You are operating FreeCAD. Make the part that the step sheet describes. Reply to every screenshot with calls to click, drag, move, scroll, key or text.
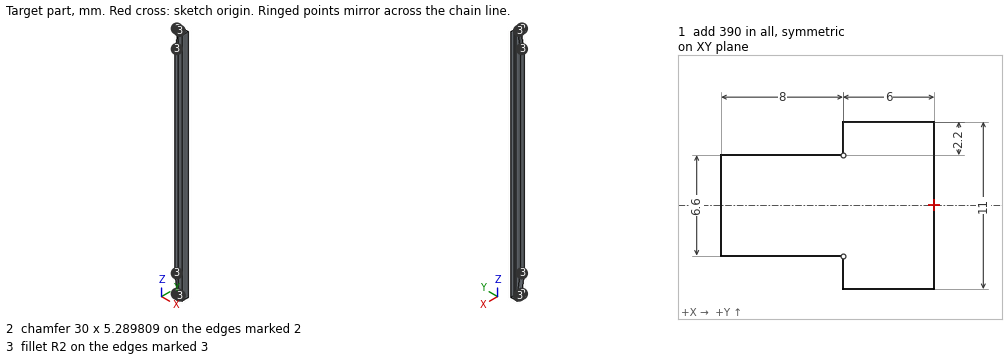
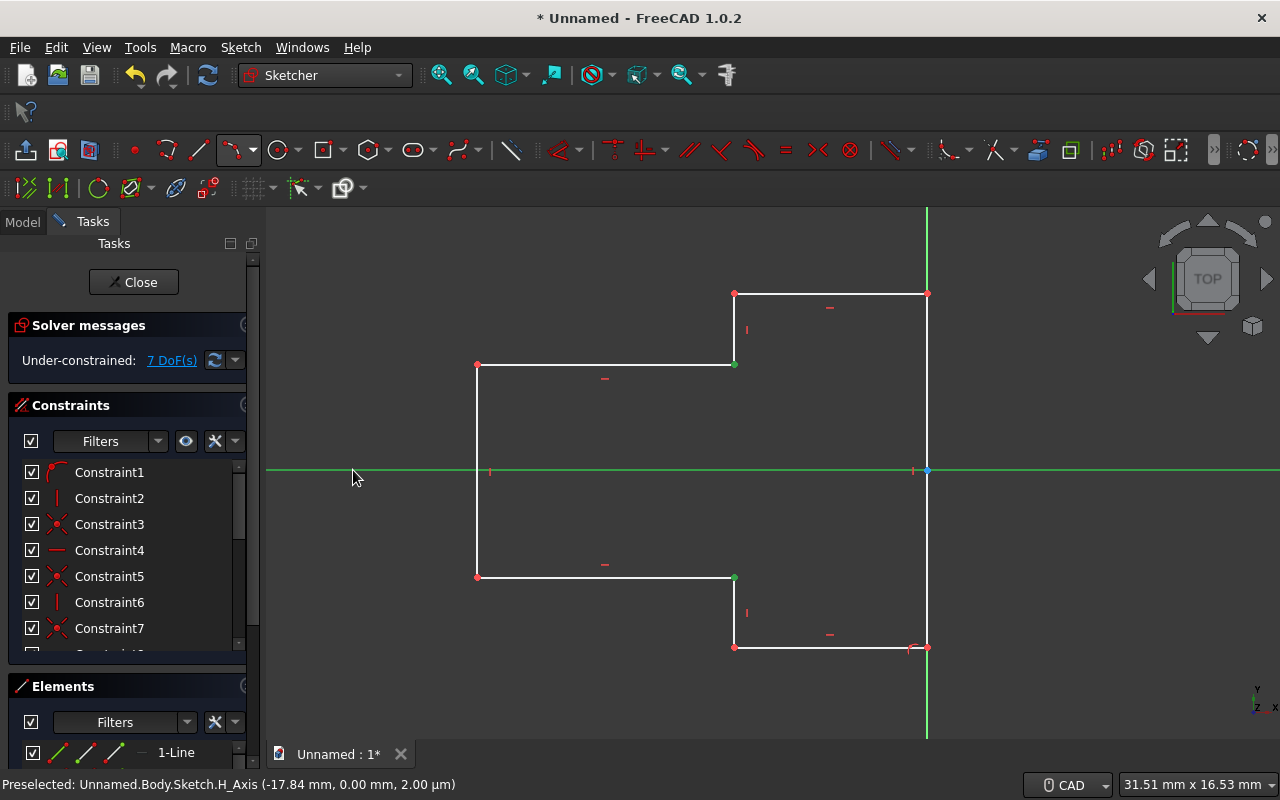
click(818, 150)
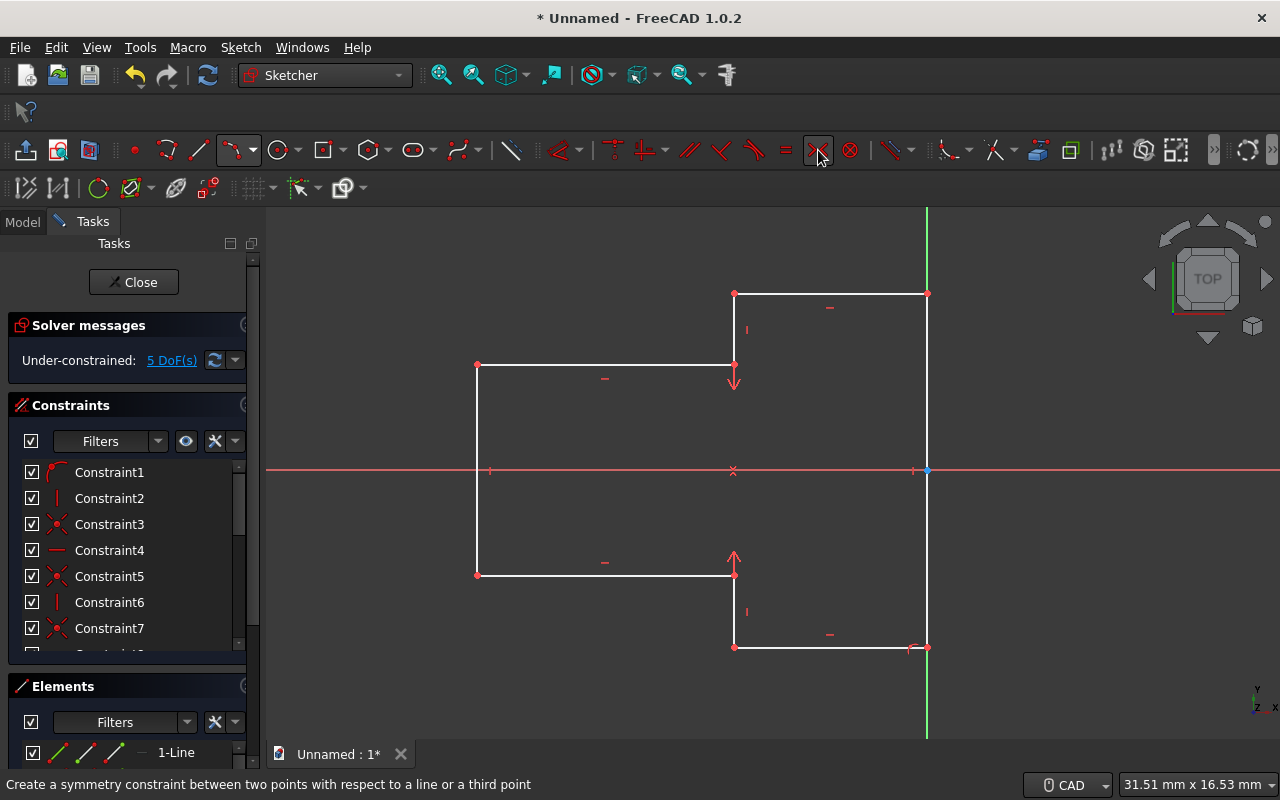
click(558, 150)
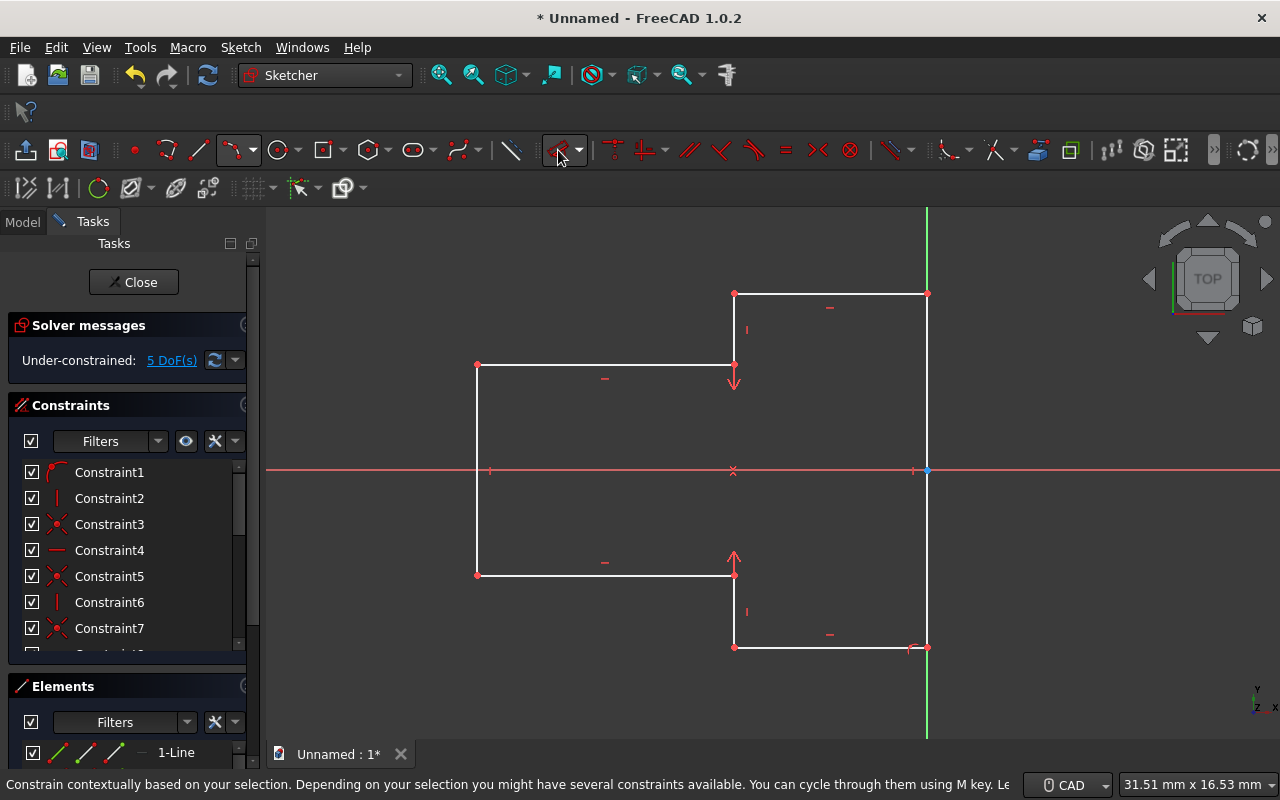
click(869, 294)
click(831, 260)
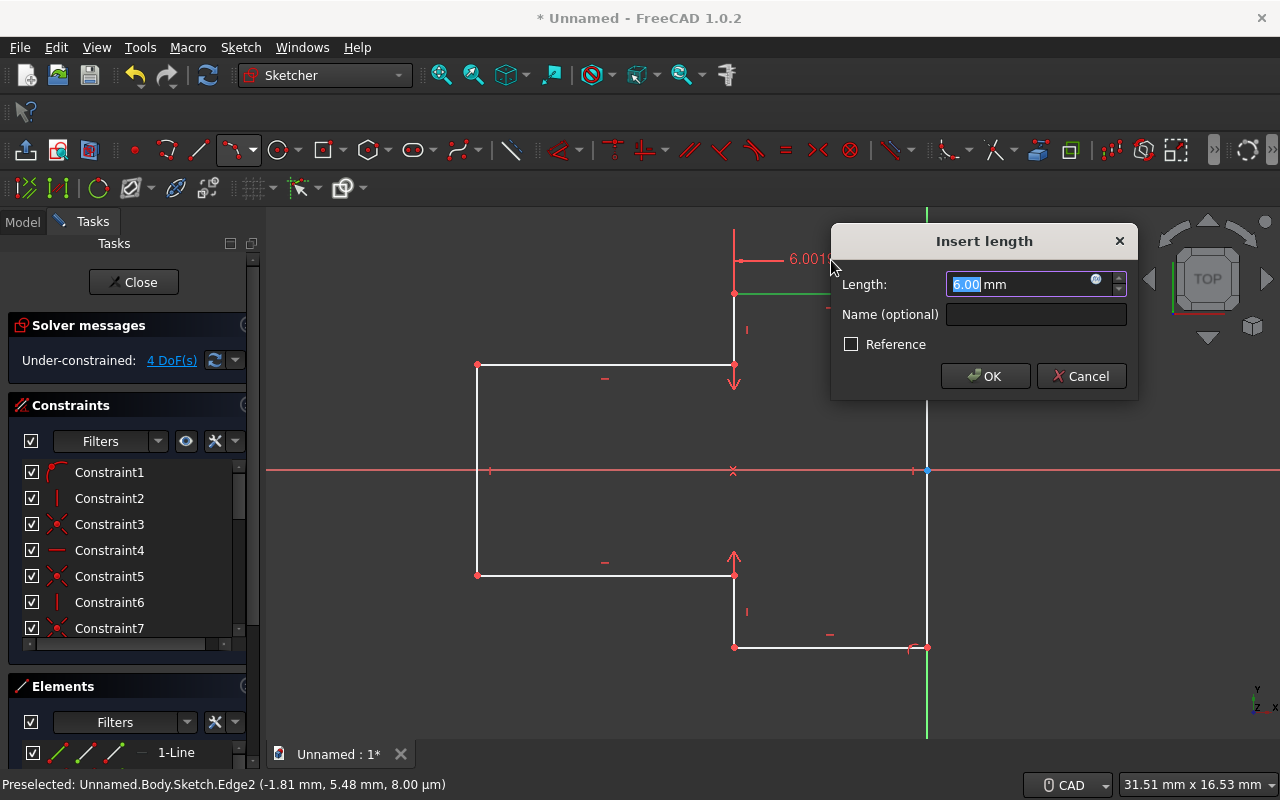
text(6)
key(Return)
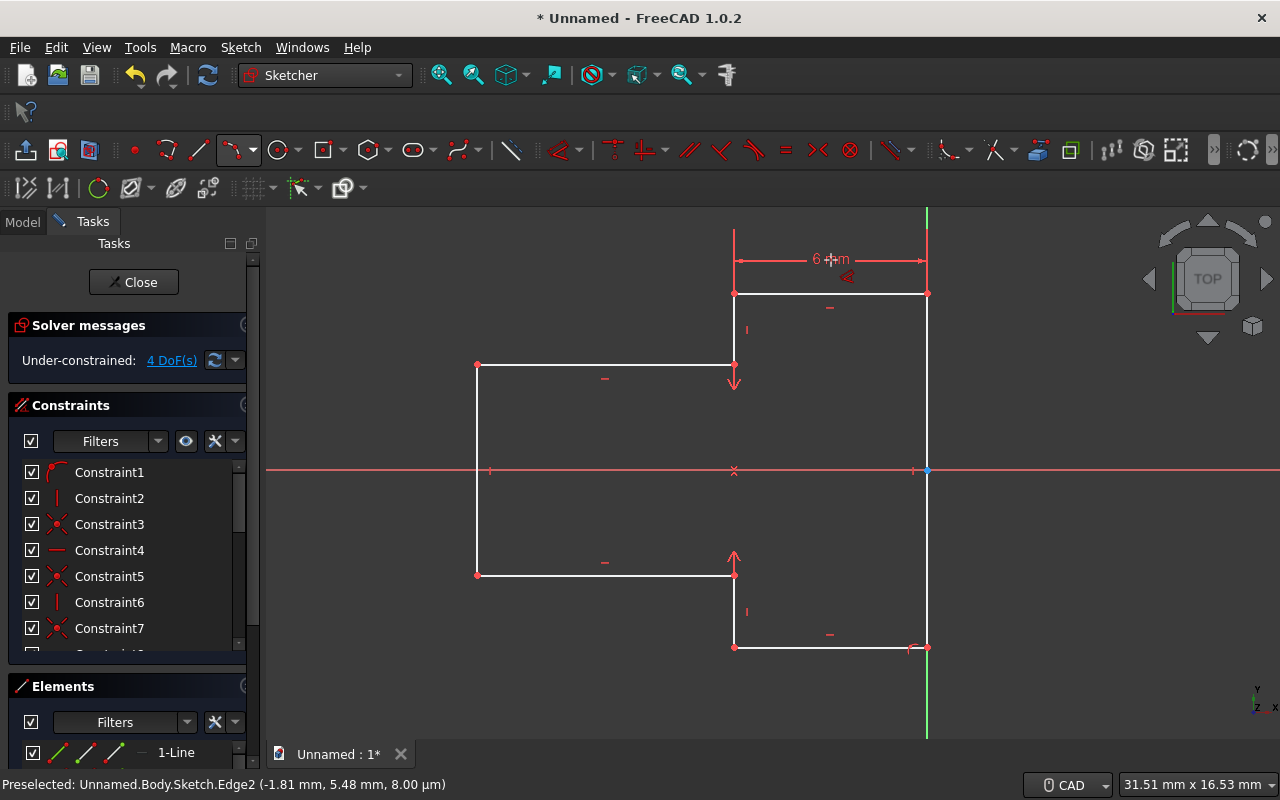
click(657, 365)
click(606, 331)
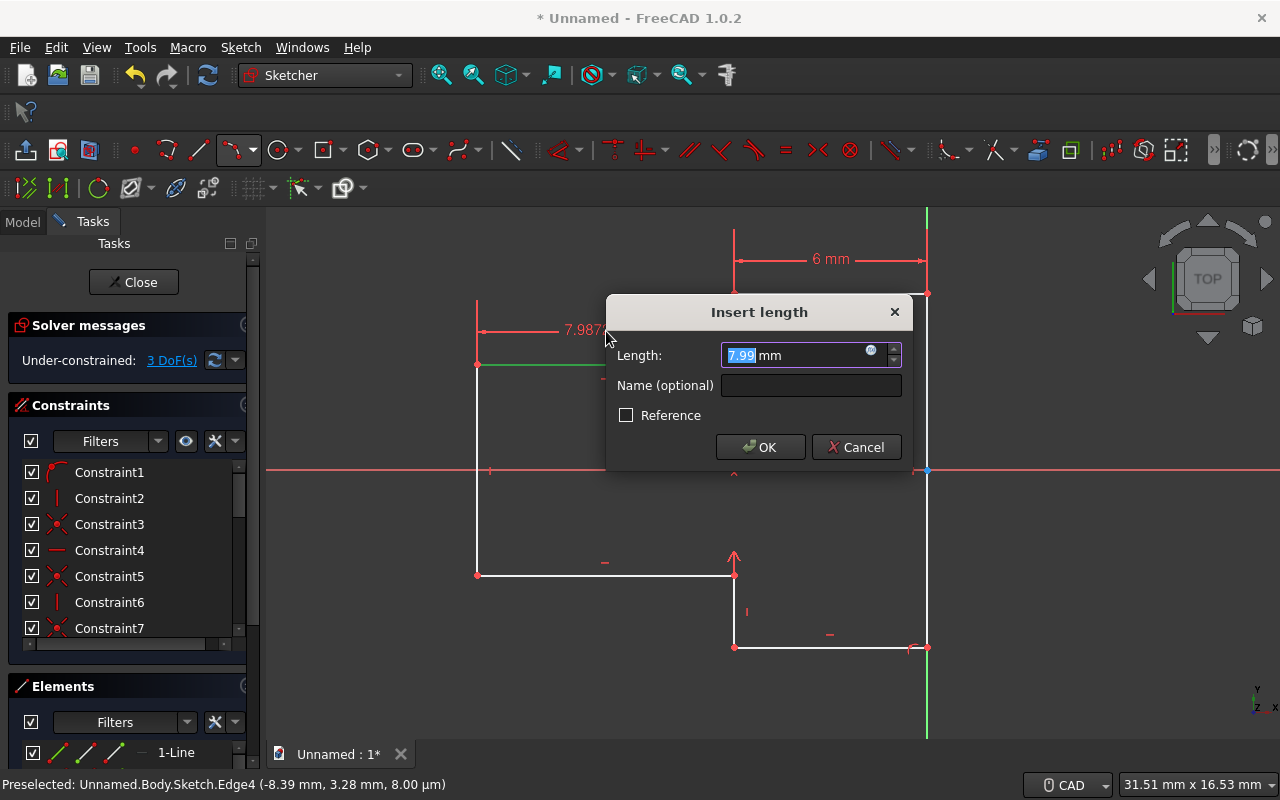
text(8)
key(Return)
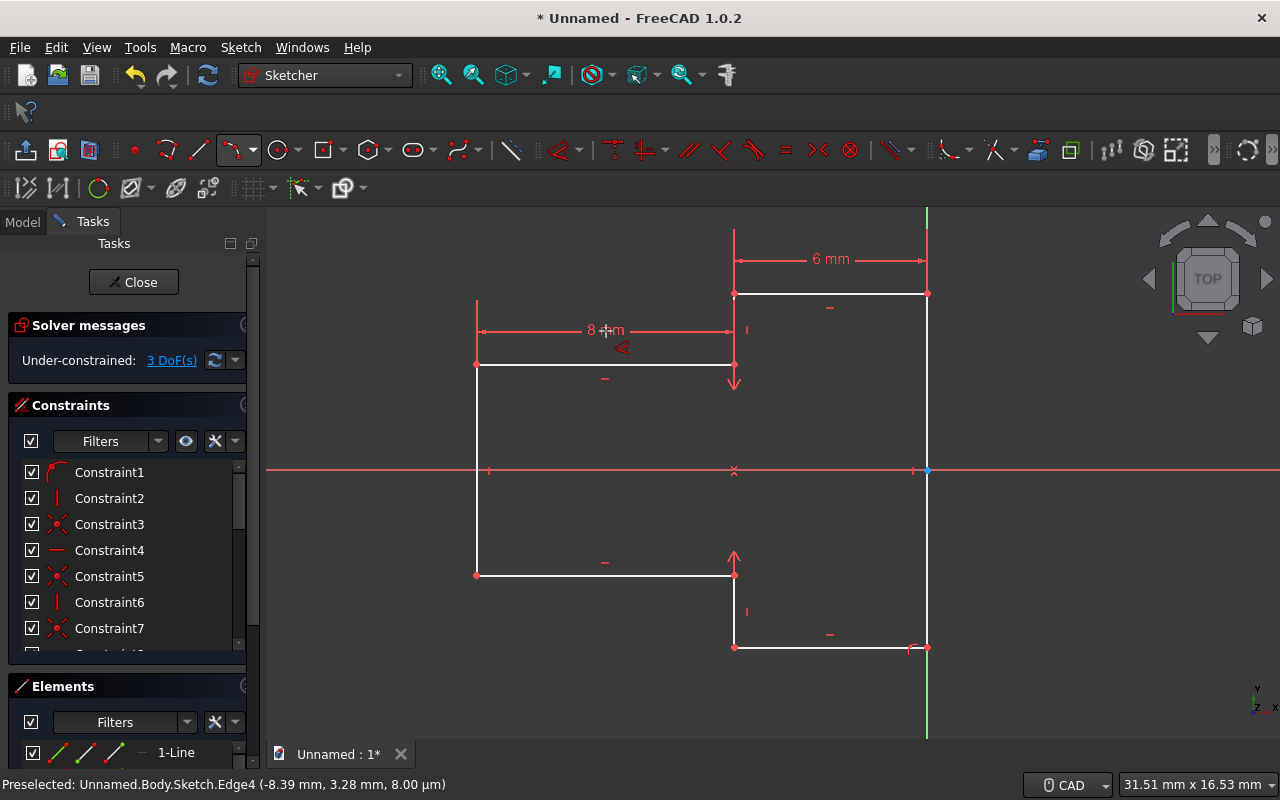
click(927, 542)
click(961, 390)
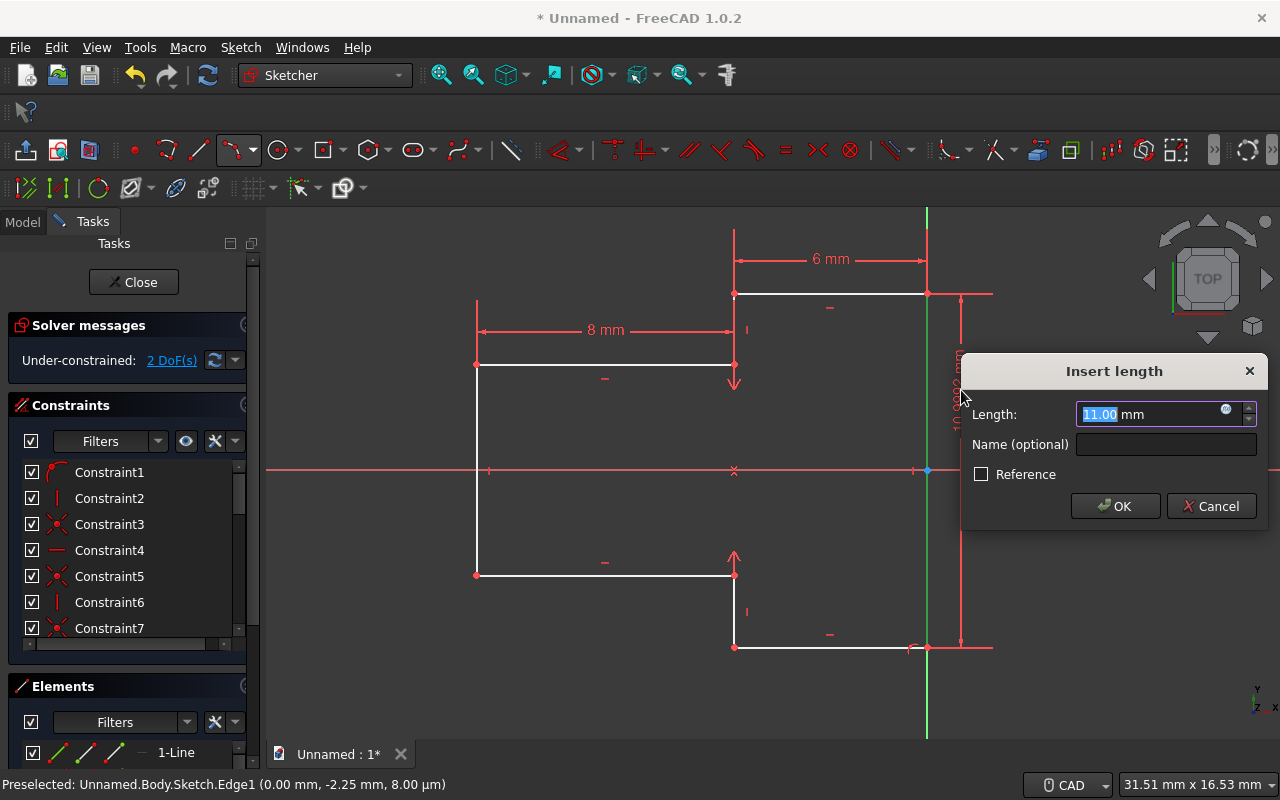
text(11)
key(Return)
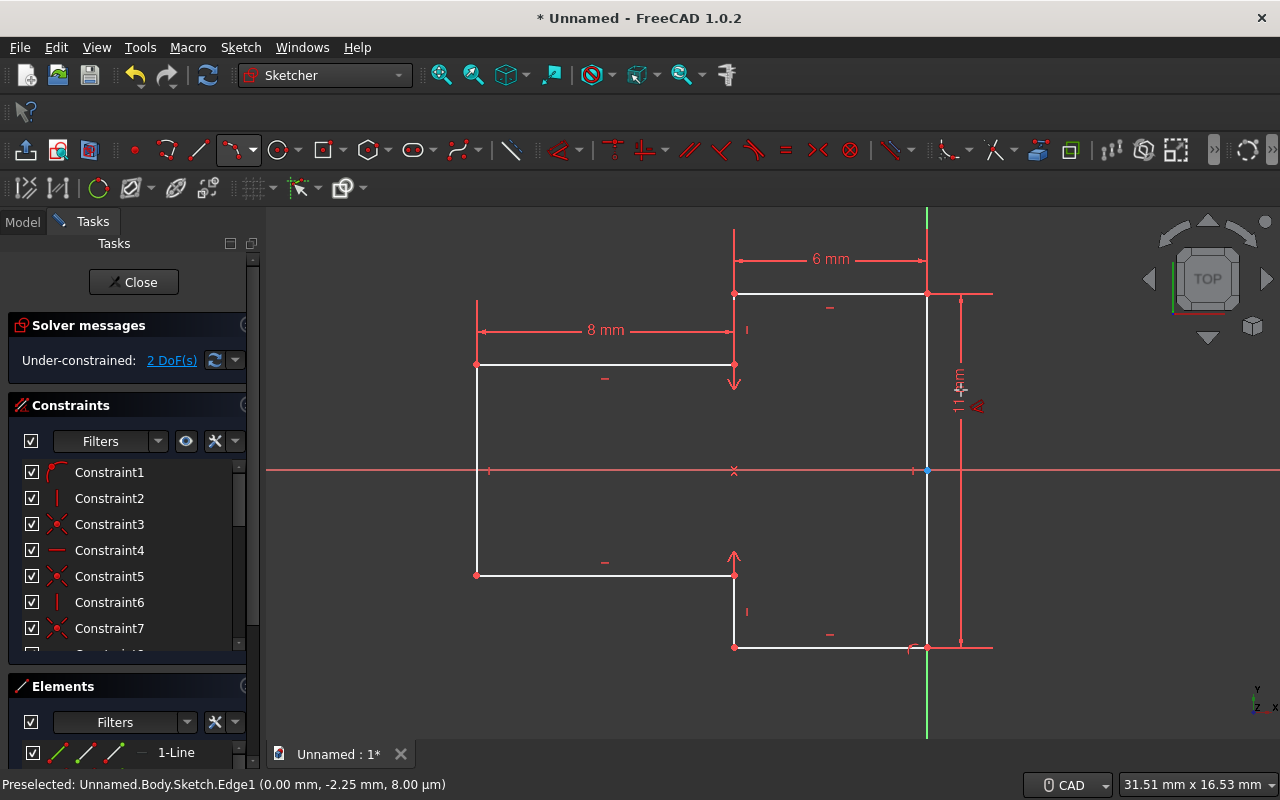
click(734, 315)
click(768, 329)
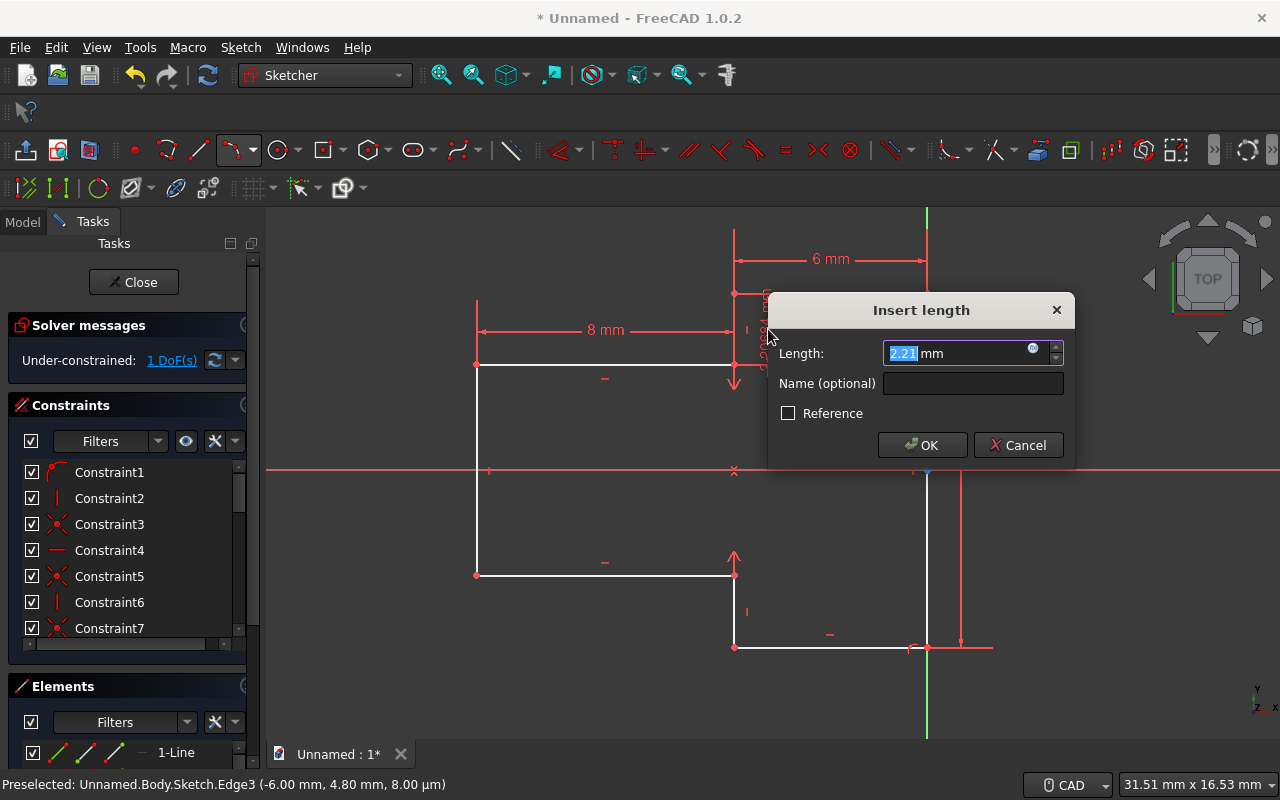
text(2.2)
key(Return)